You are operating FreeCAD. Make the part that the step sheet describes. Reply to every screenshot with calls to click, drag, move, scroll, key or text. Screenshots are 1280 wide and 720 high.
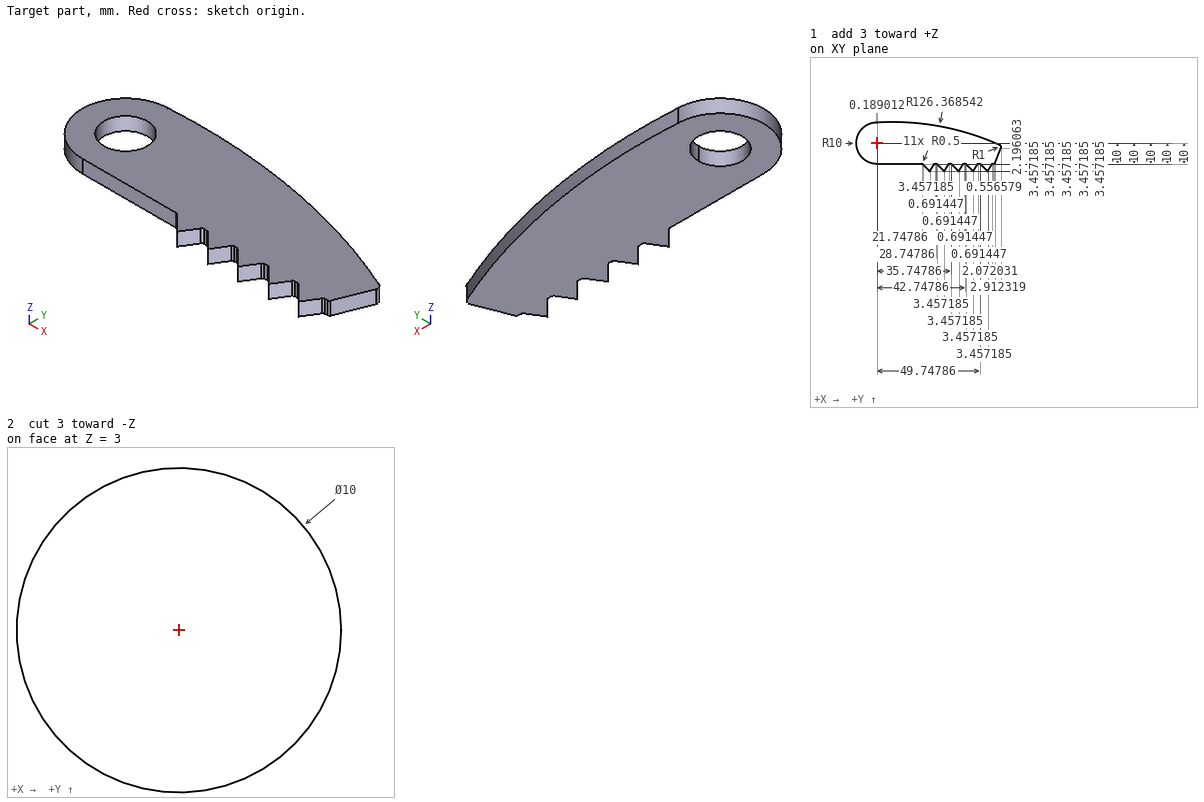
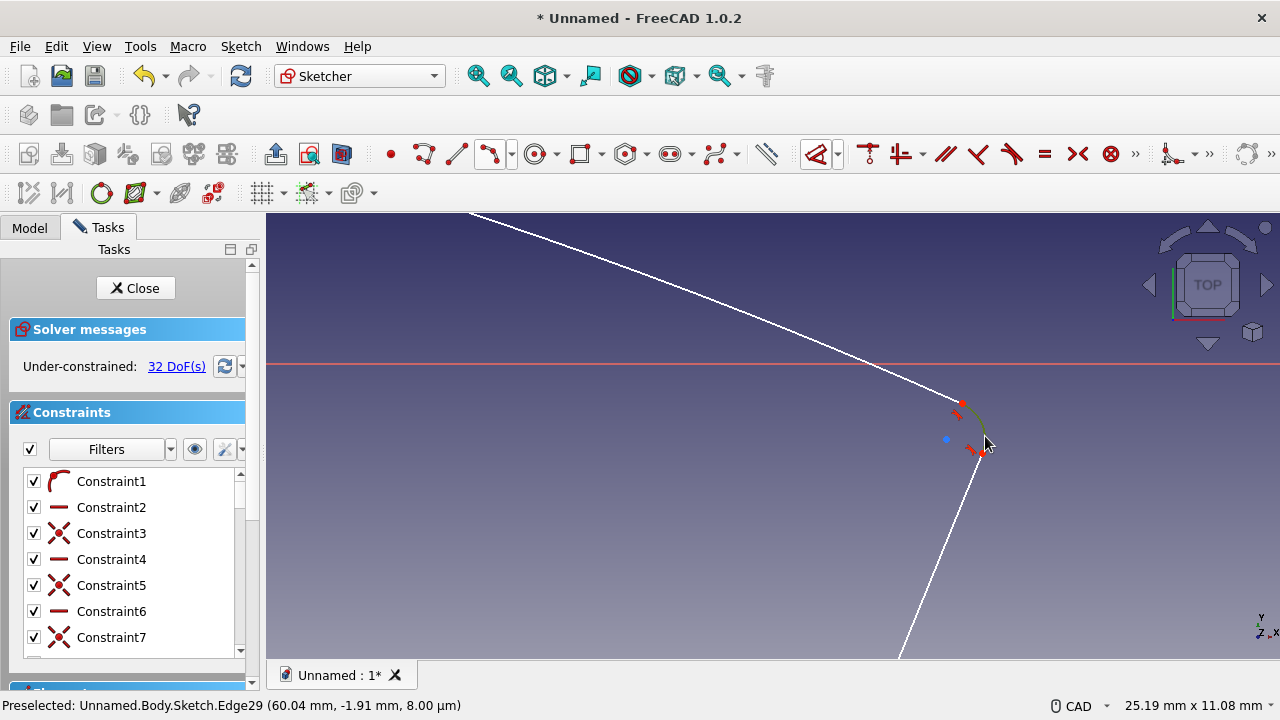
key(k)
key(r)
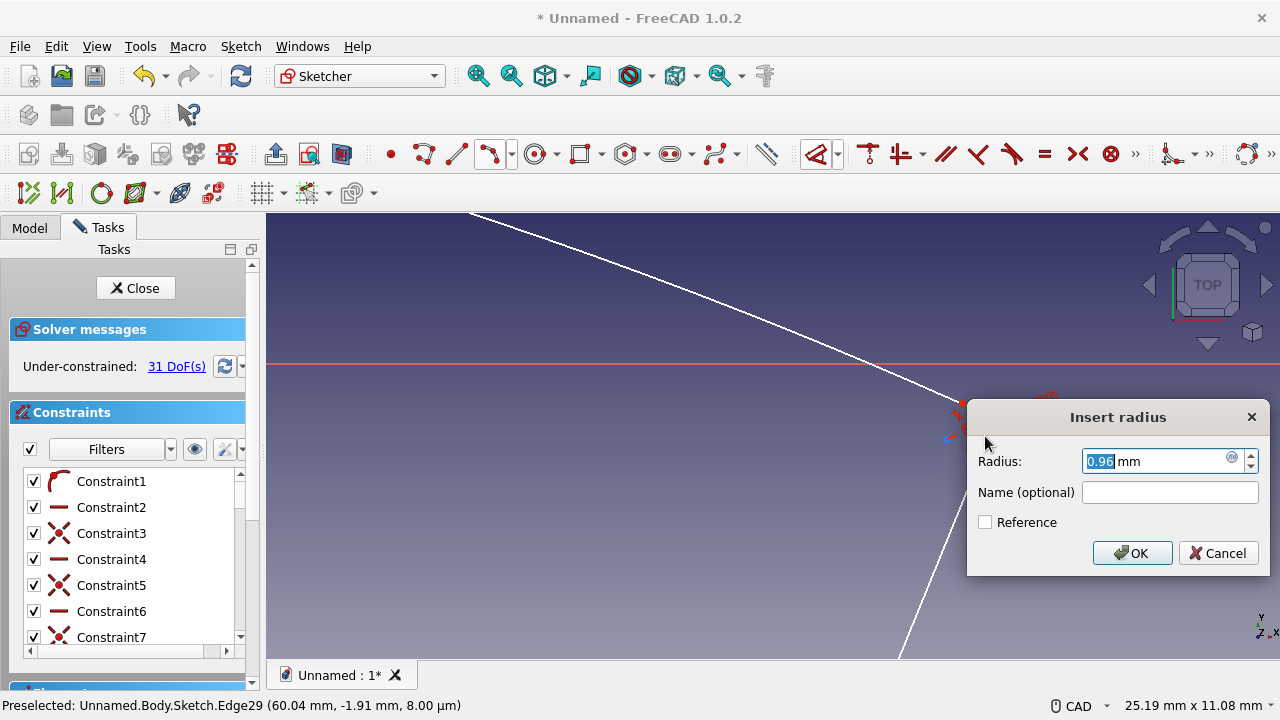
text(1)
key(Return)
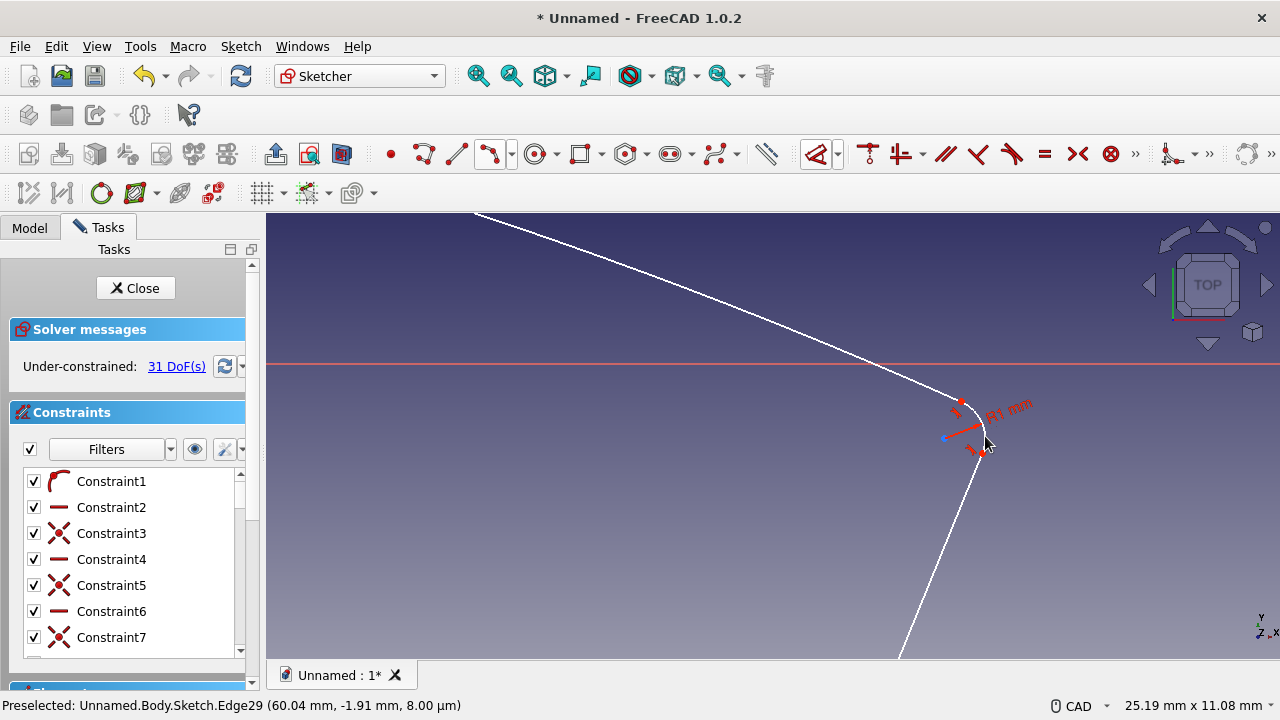
scroll(990, 436, down, 8)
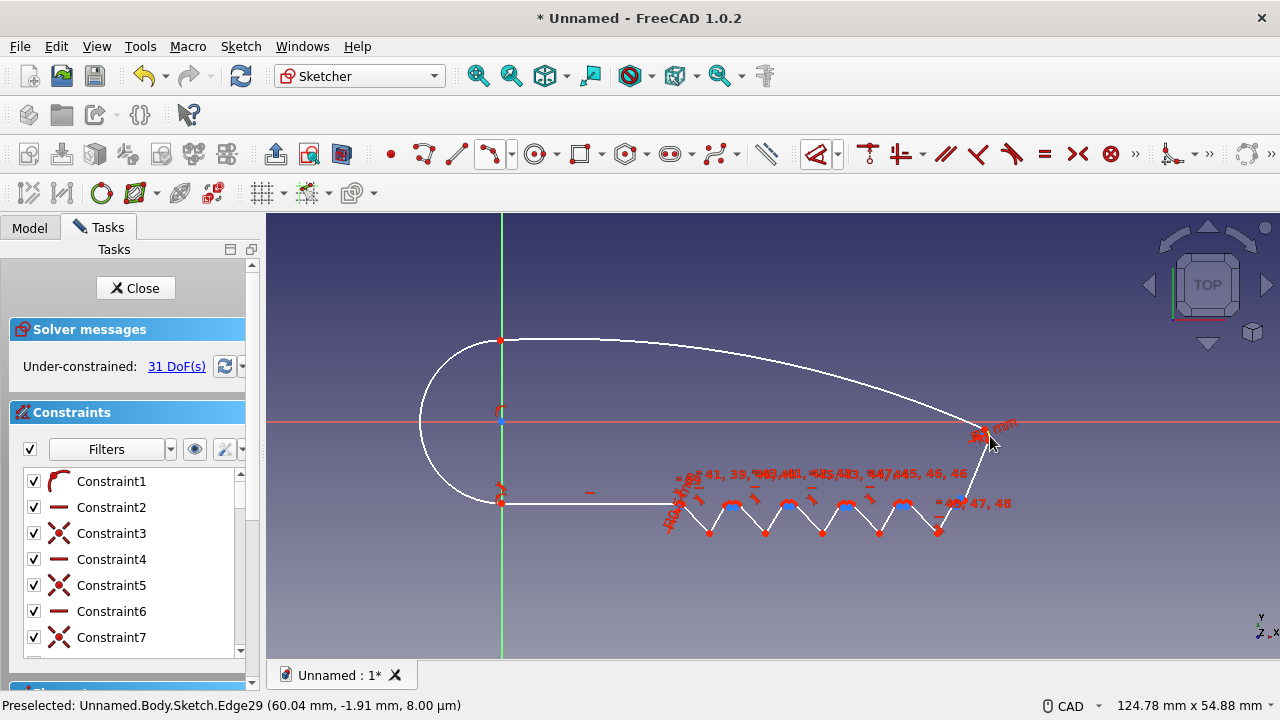
click(845, 379)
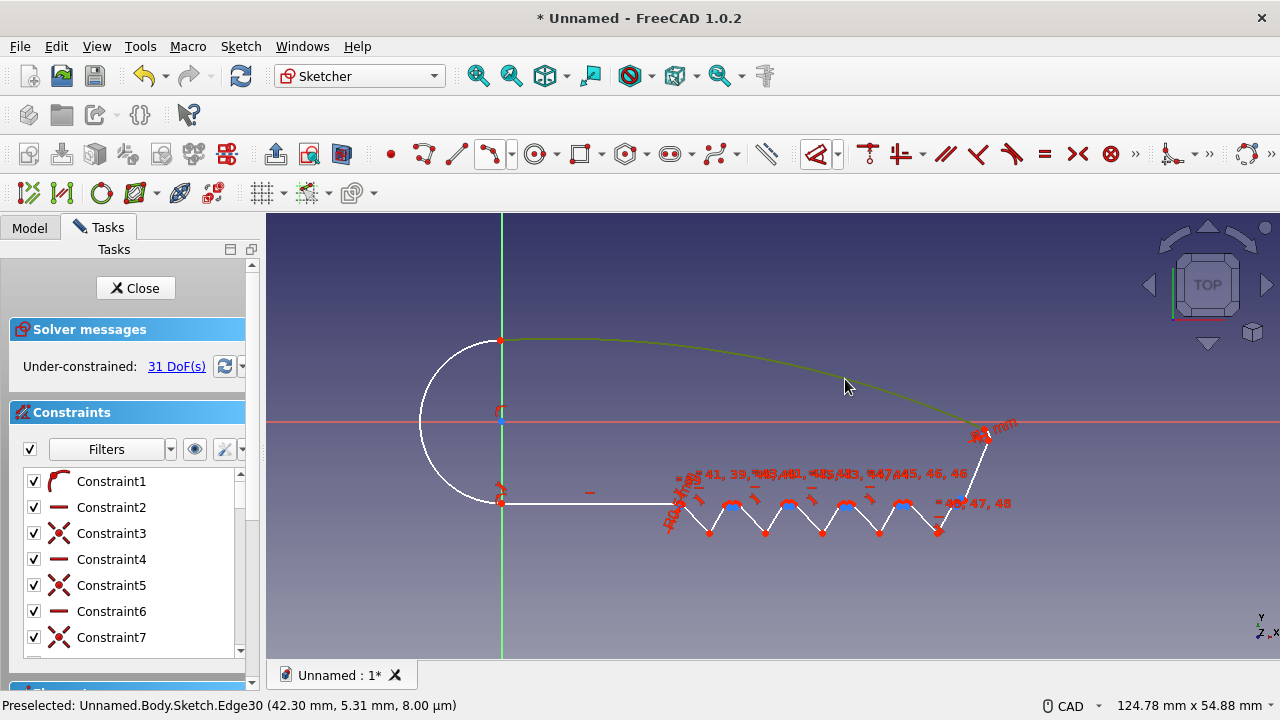
click(838, 154)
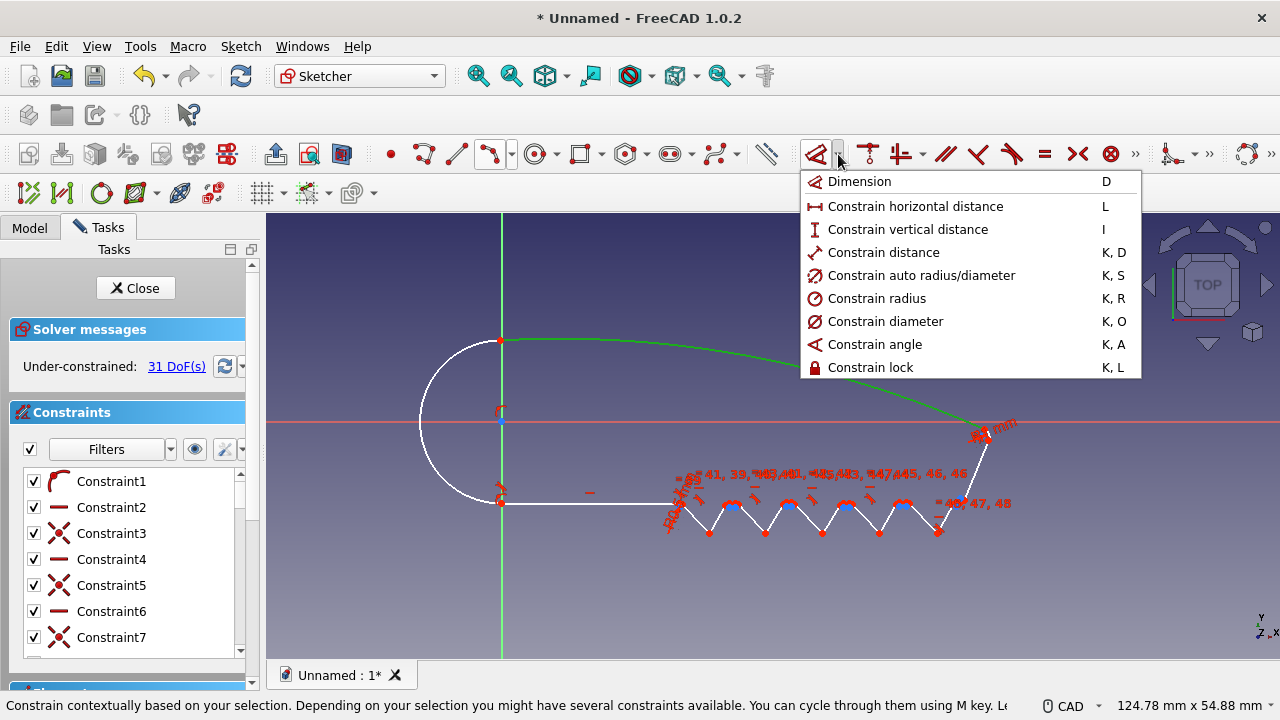
click(971, 298)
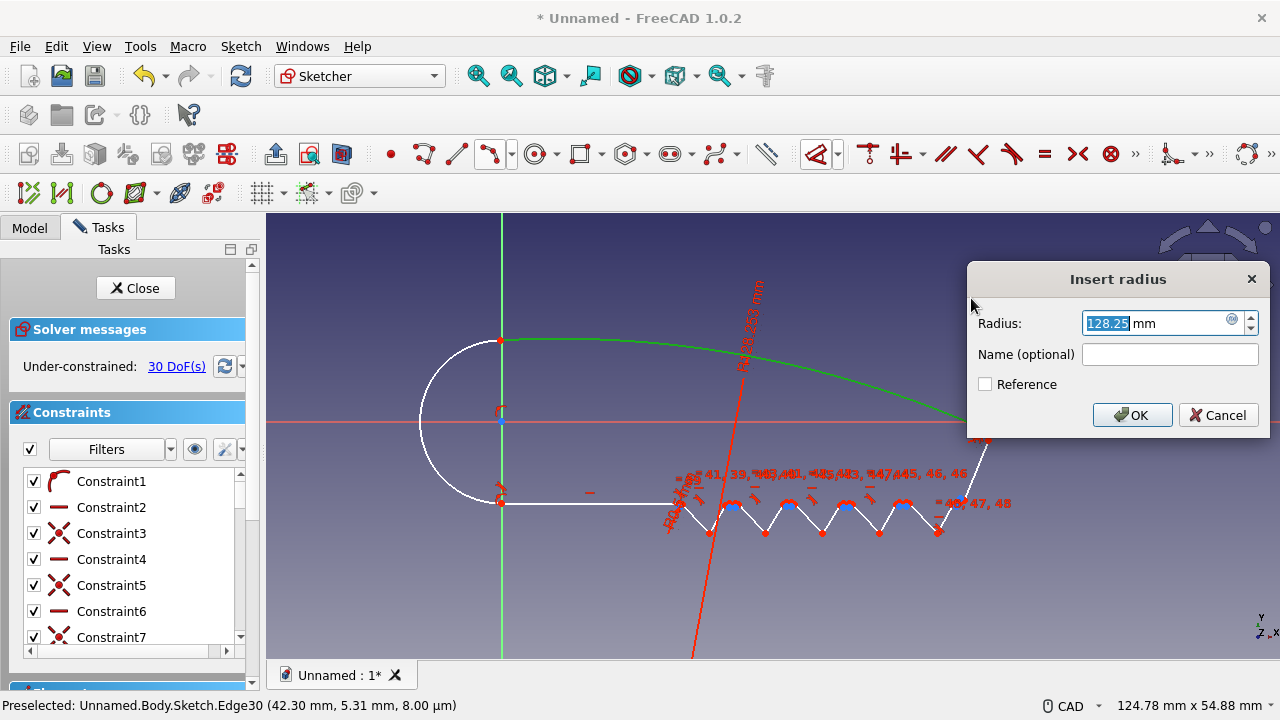
text(126.368542)
key(Return)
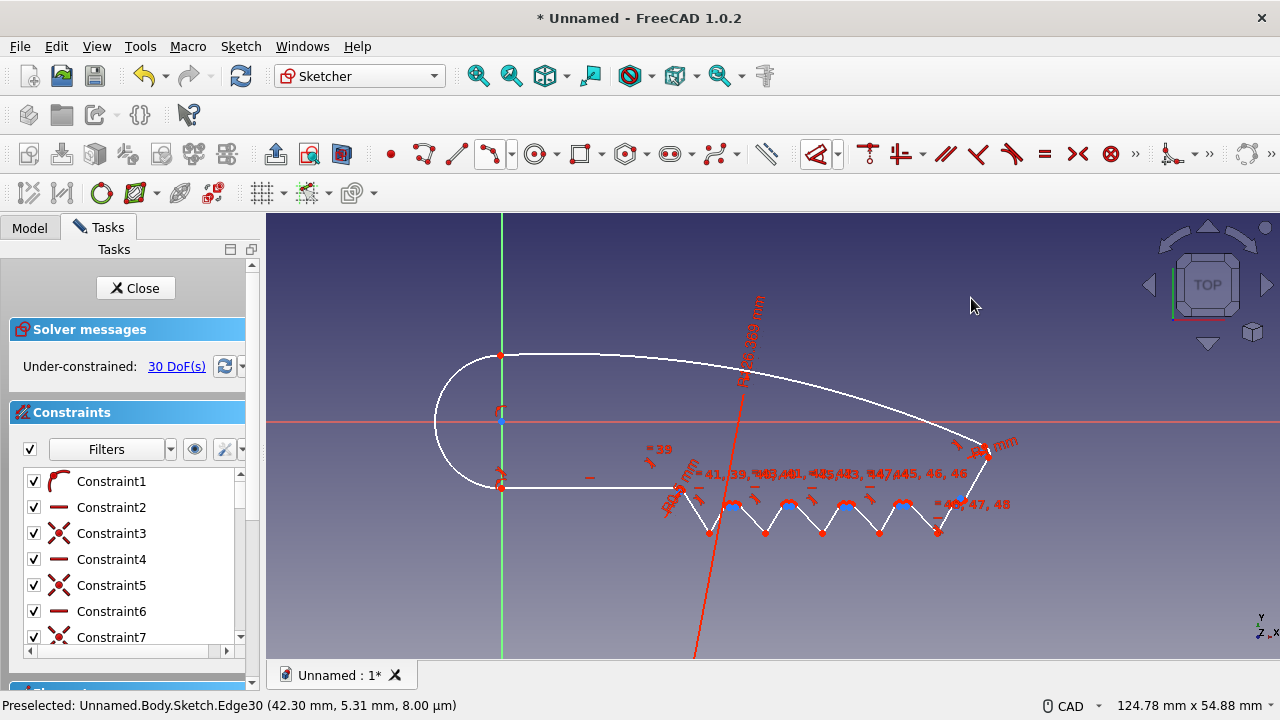
click(447, 384)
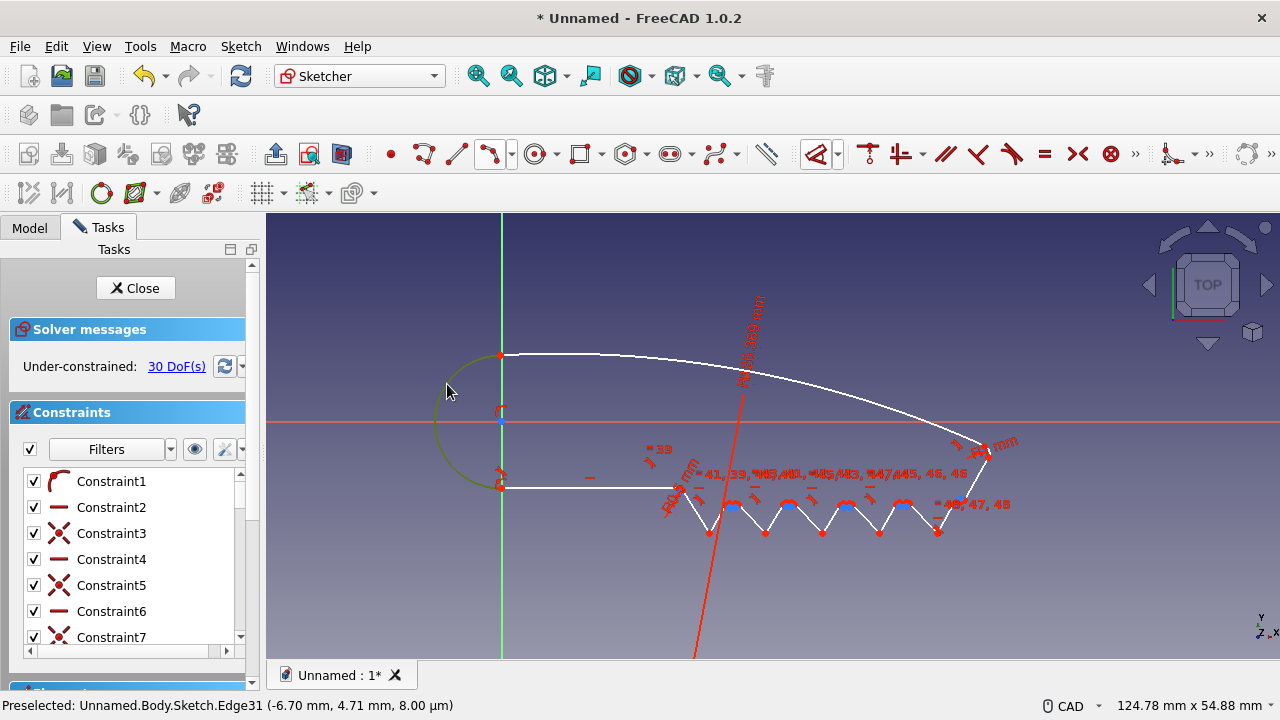
click(838, 154)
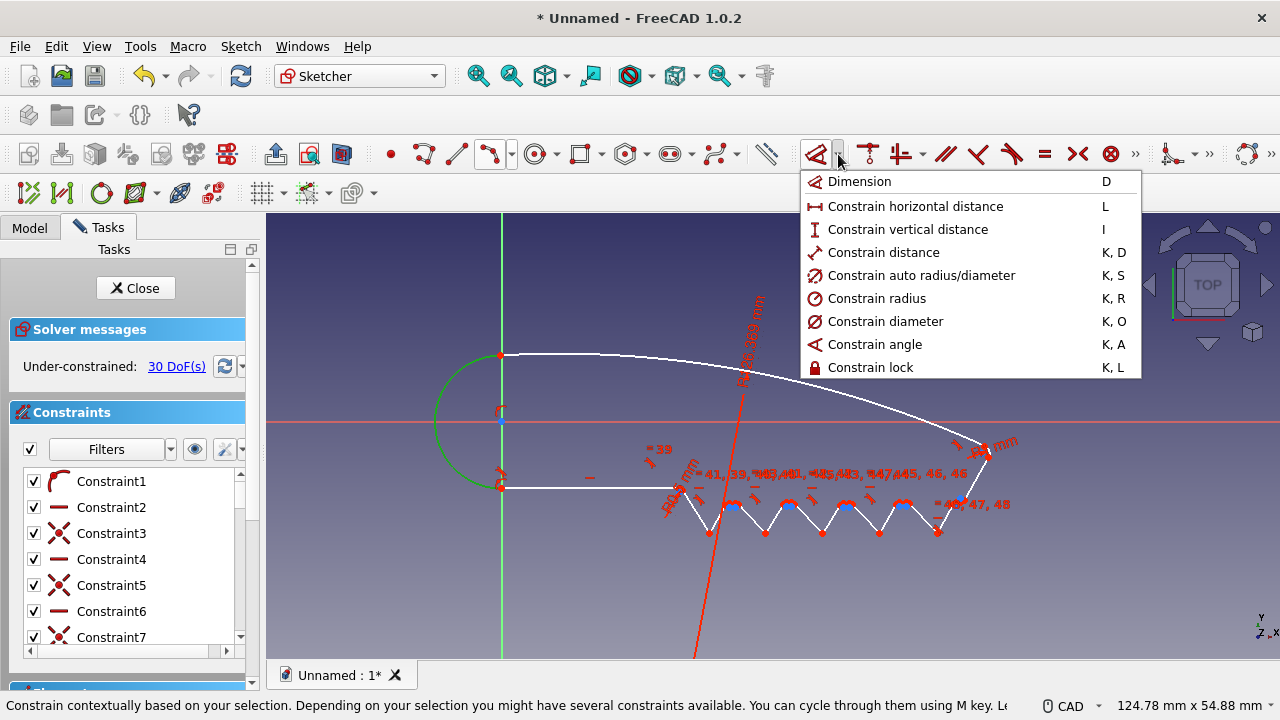
click(971, 298)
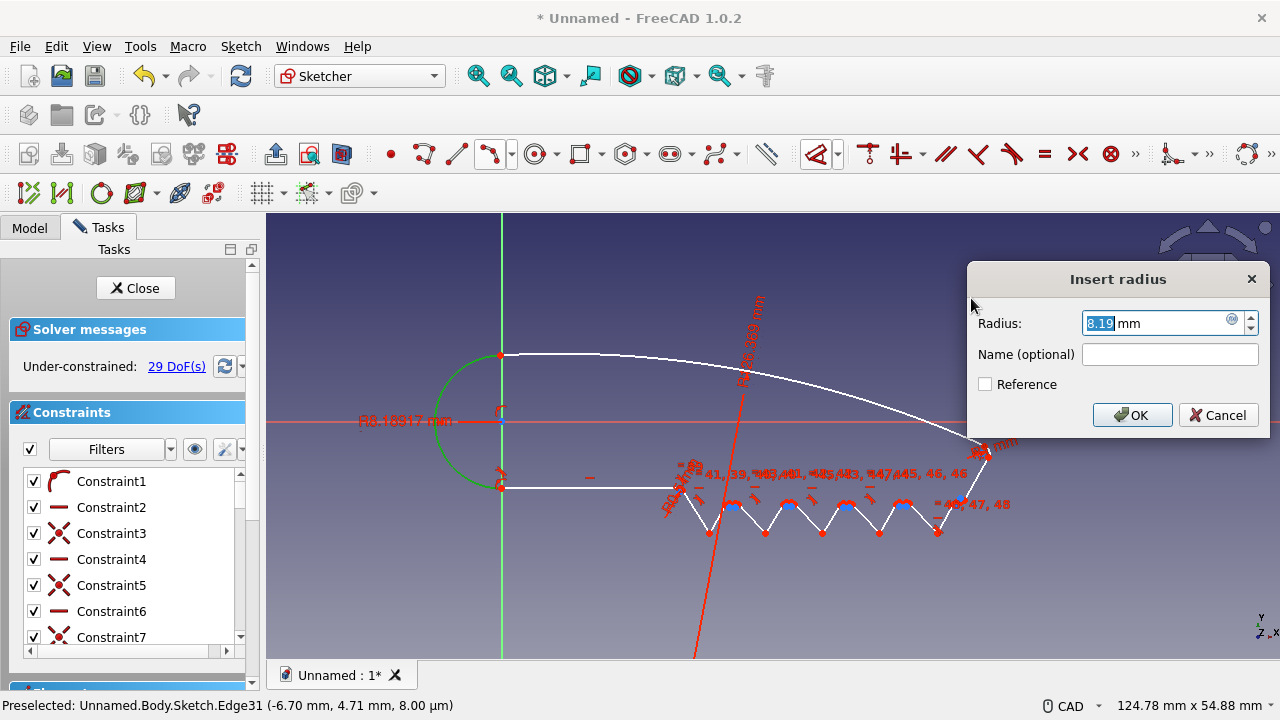
text(10)
key(Return)